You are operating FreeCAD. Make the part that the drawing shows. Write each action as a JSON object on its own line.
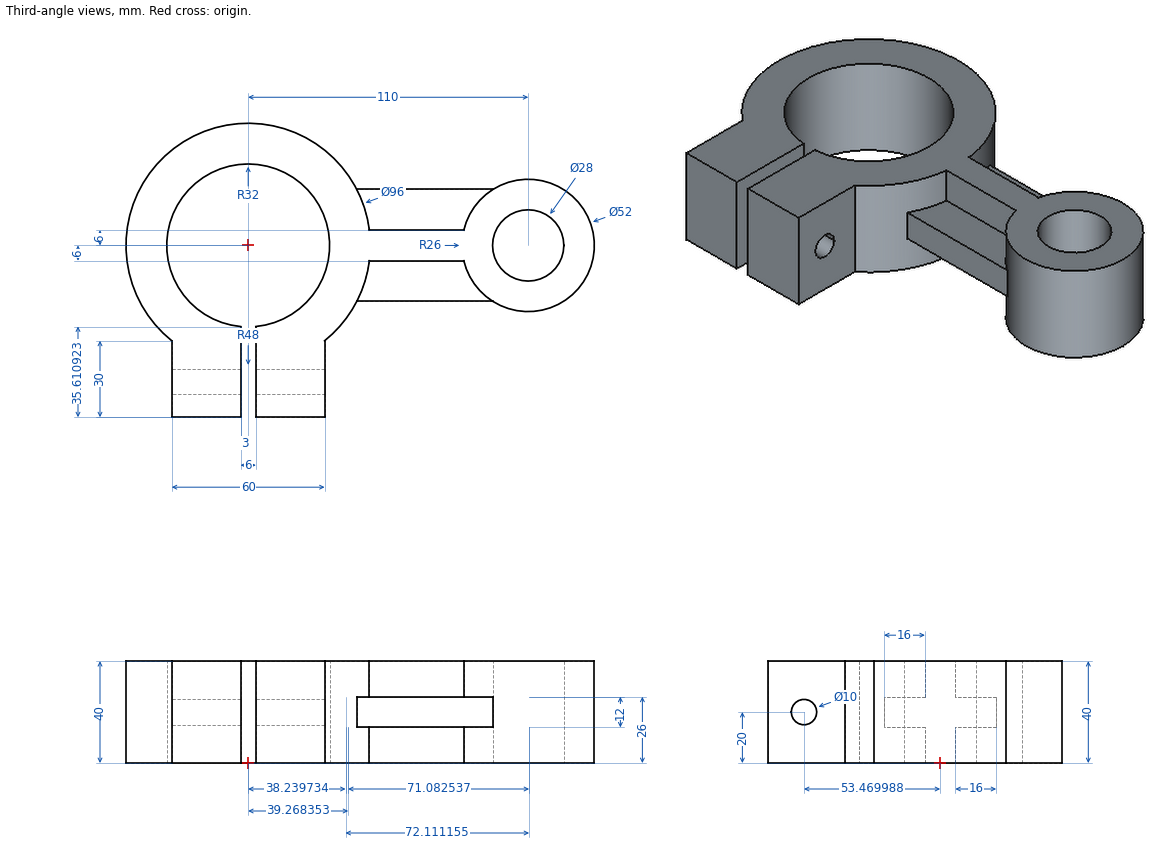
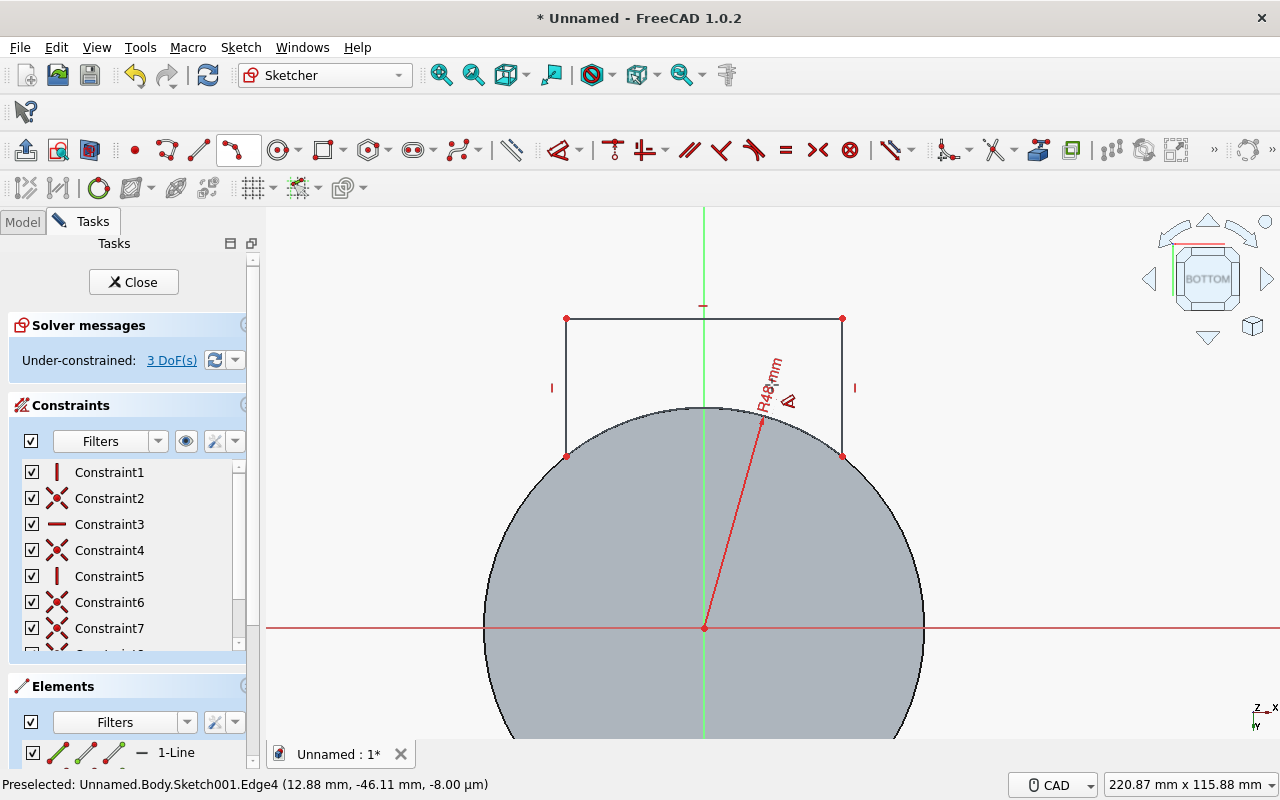
{"action": "left_click", "coordinate": [566, 415]}
{"action": "left_click", "coordinate": [532, 388]}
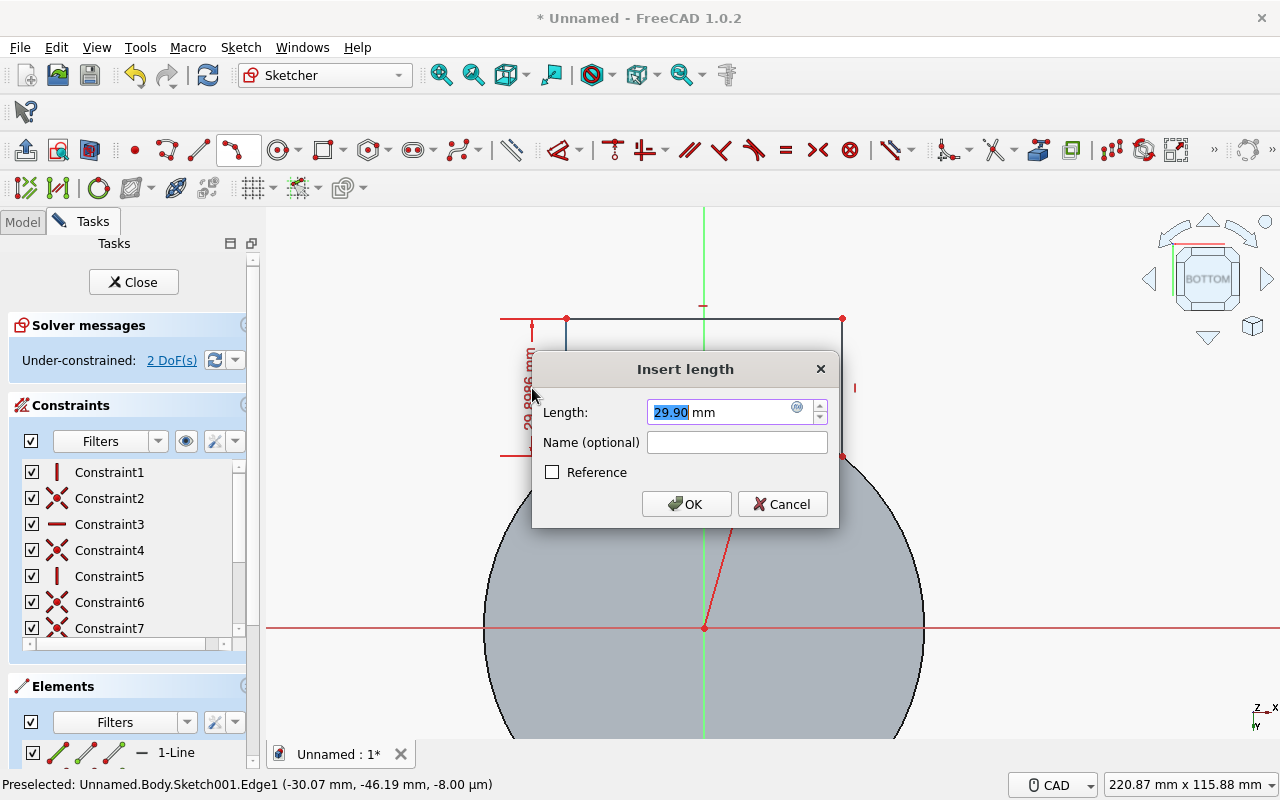
{"action": "type", "text": "30"}
{"action": "key", "text": "Return"}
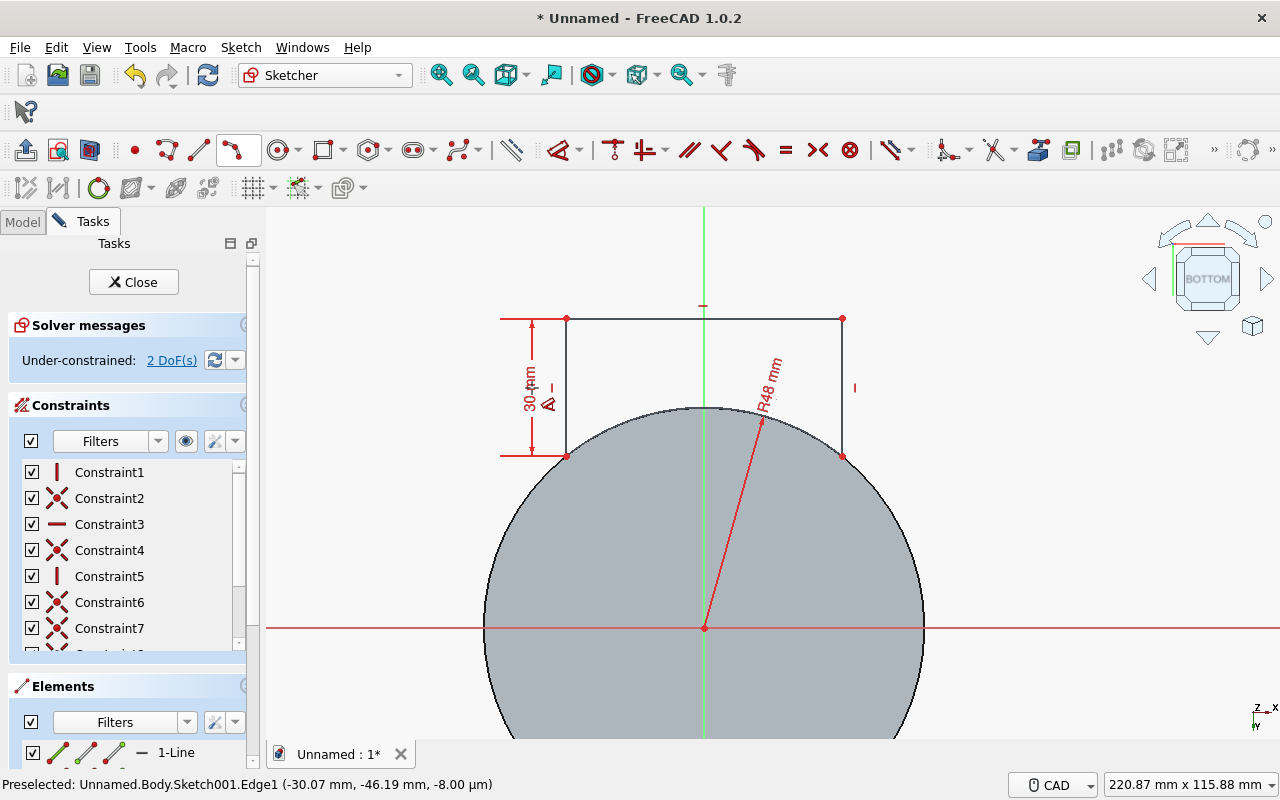
{"action": "left_click", "coordinate": [649, 319]}
{"action": "left_click", "coordinate": [641, 285]}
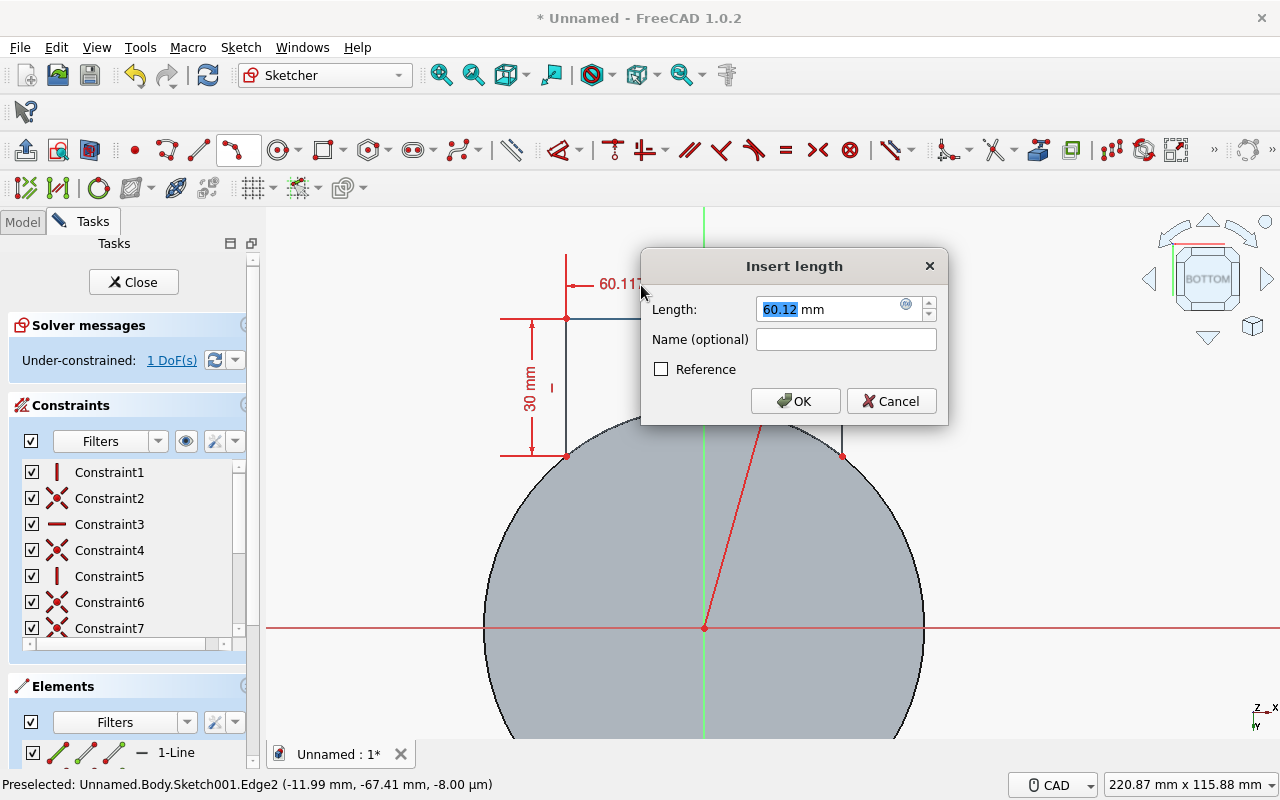
{"action": "type", "text": "60"}
{"action": "key", "text": "Return"}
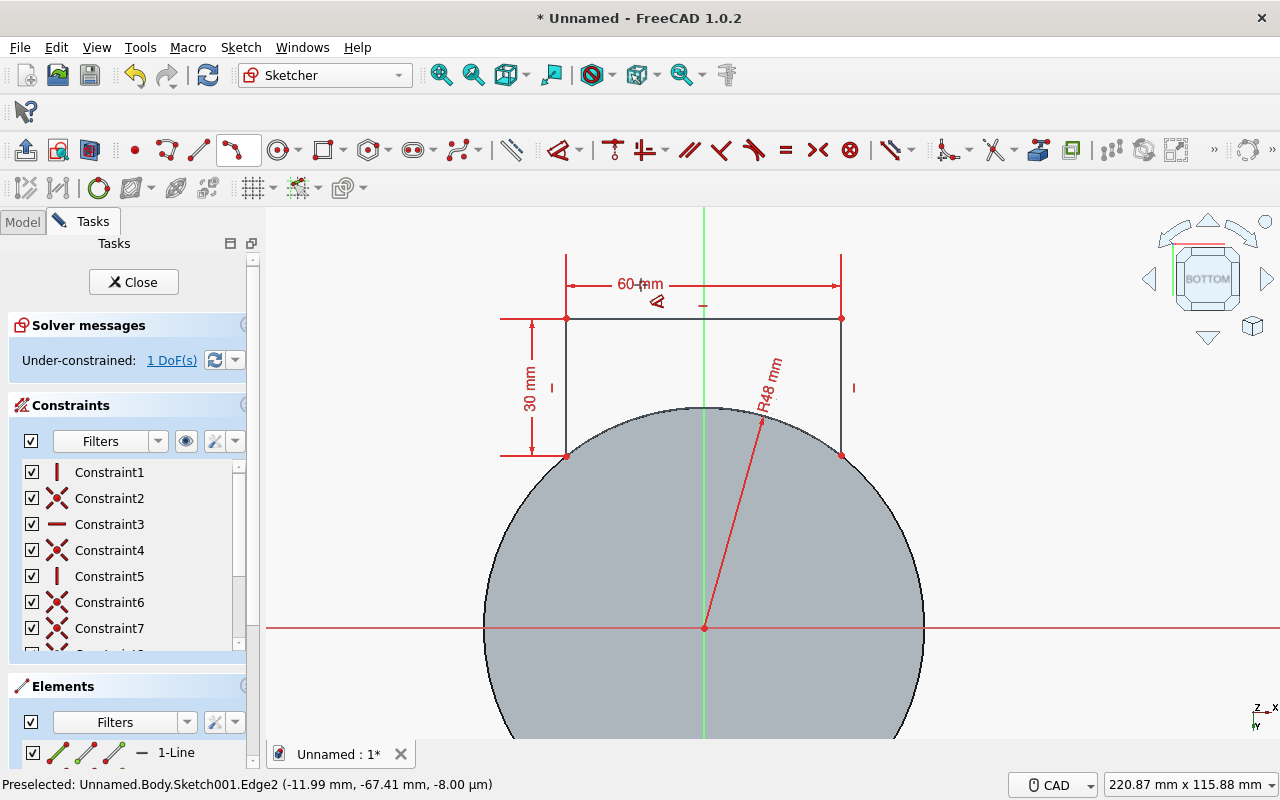
{"action": "left_click", "coordinate": [841, 360]}
{"action": "left_click", "coordinate": [875, 387]}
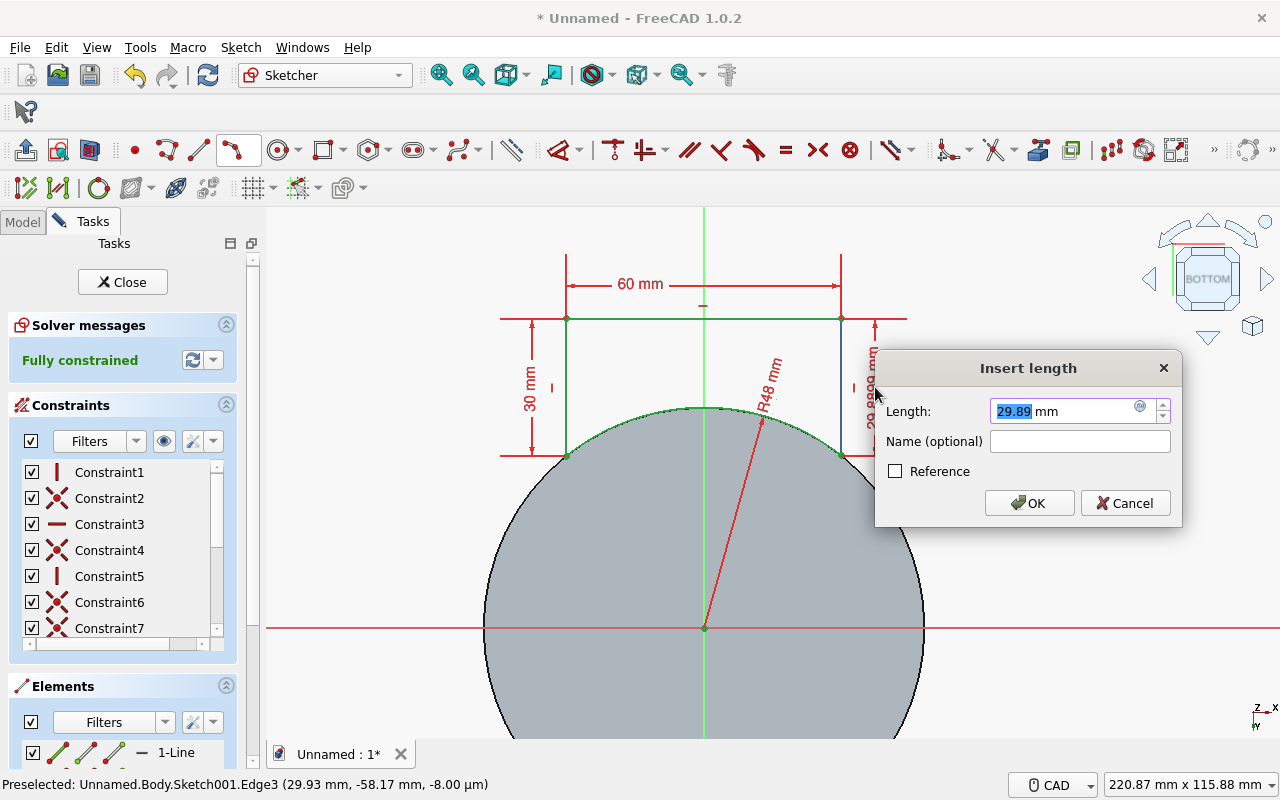
{"action": "type", "text": "30"}
{"action": "key", "text": "Return"}
{"action": "key", "text": "Escape"}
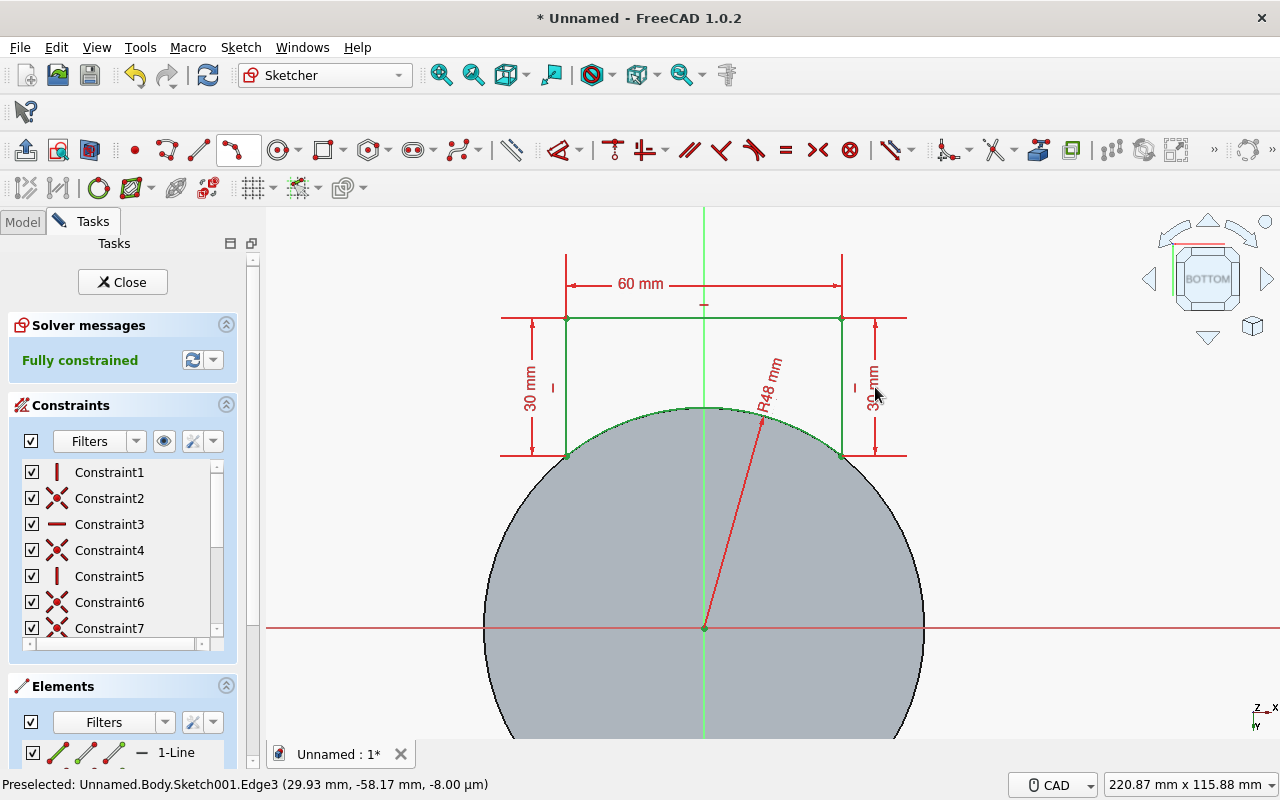
{"action": "left_click", "coordinate": [123, 282]}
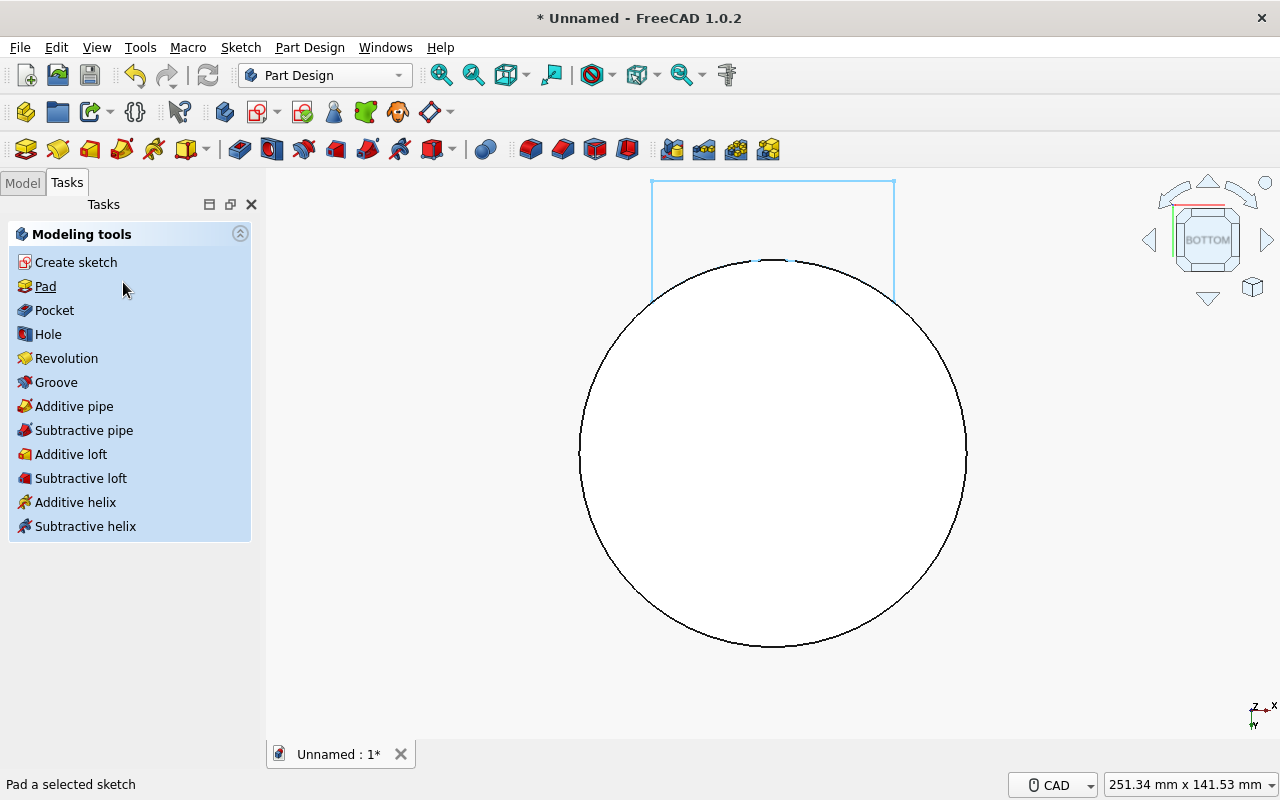
{"action": "left_click", "coordinate": [26, 150]}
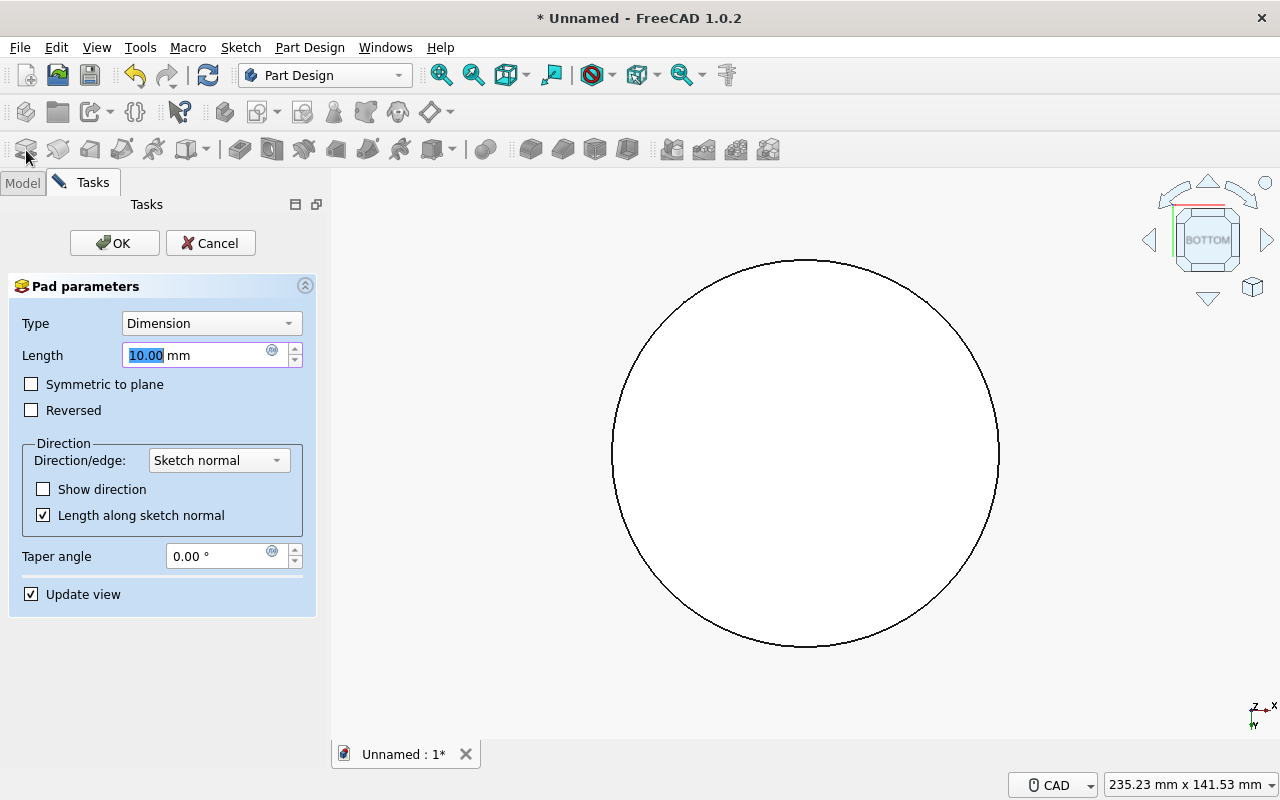
{"action": "type", "text": "40"}
{"action": "key", "text": "Tab"}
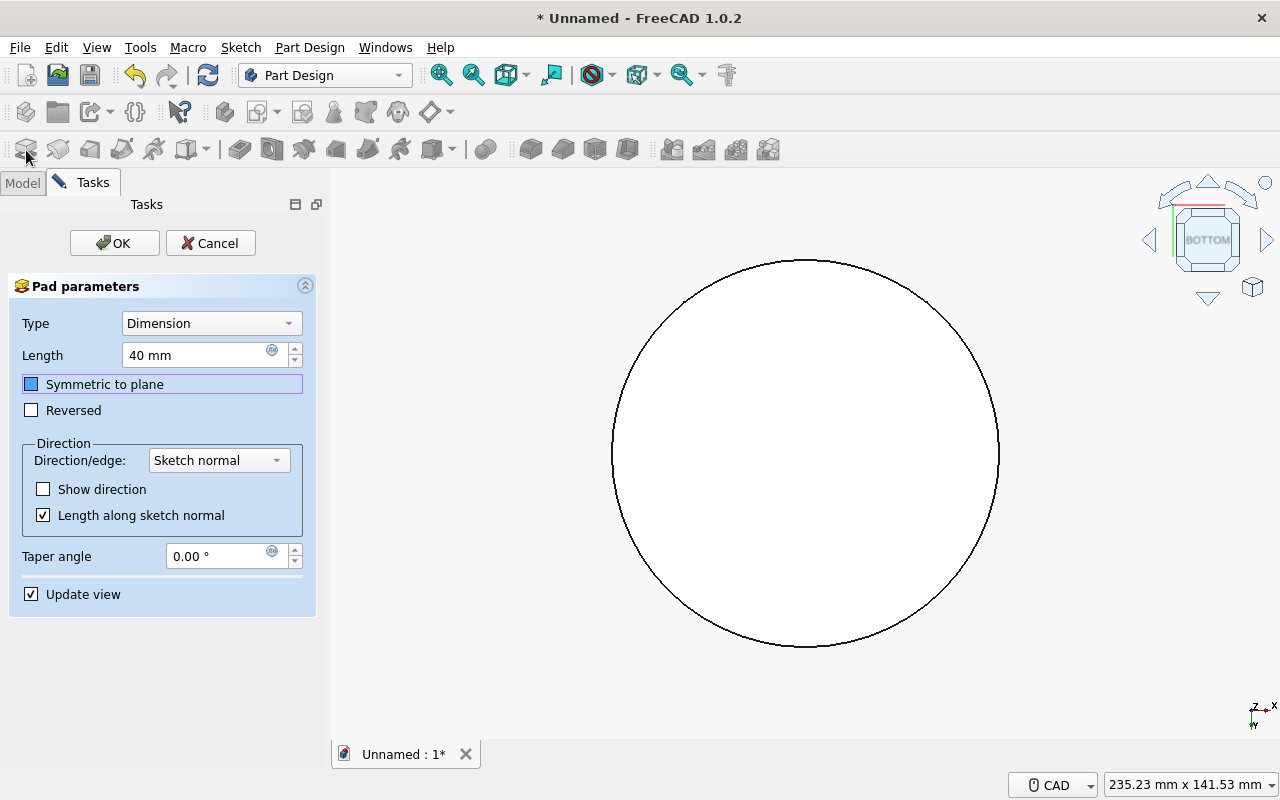
{"action": "left_click", "coordinate": [30, 410]}